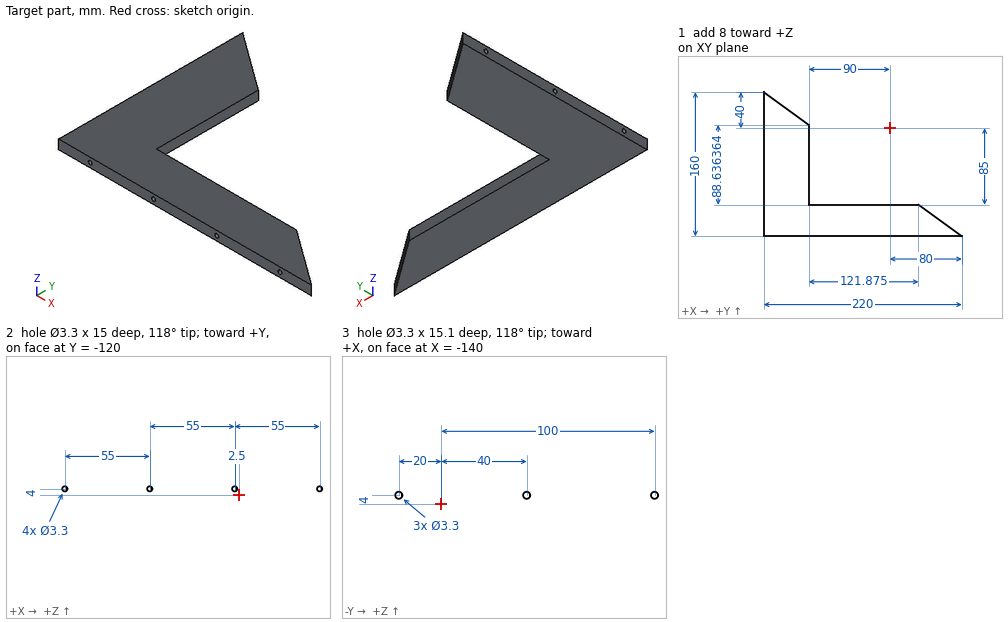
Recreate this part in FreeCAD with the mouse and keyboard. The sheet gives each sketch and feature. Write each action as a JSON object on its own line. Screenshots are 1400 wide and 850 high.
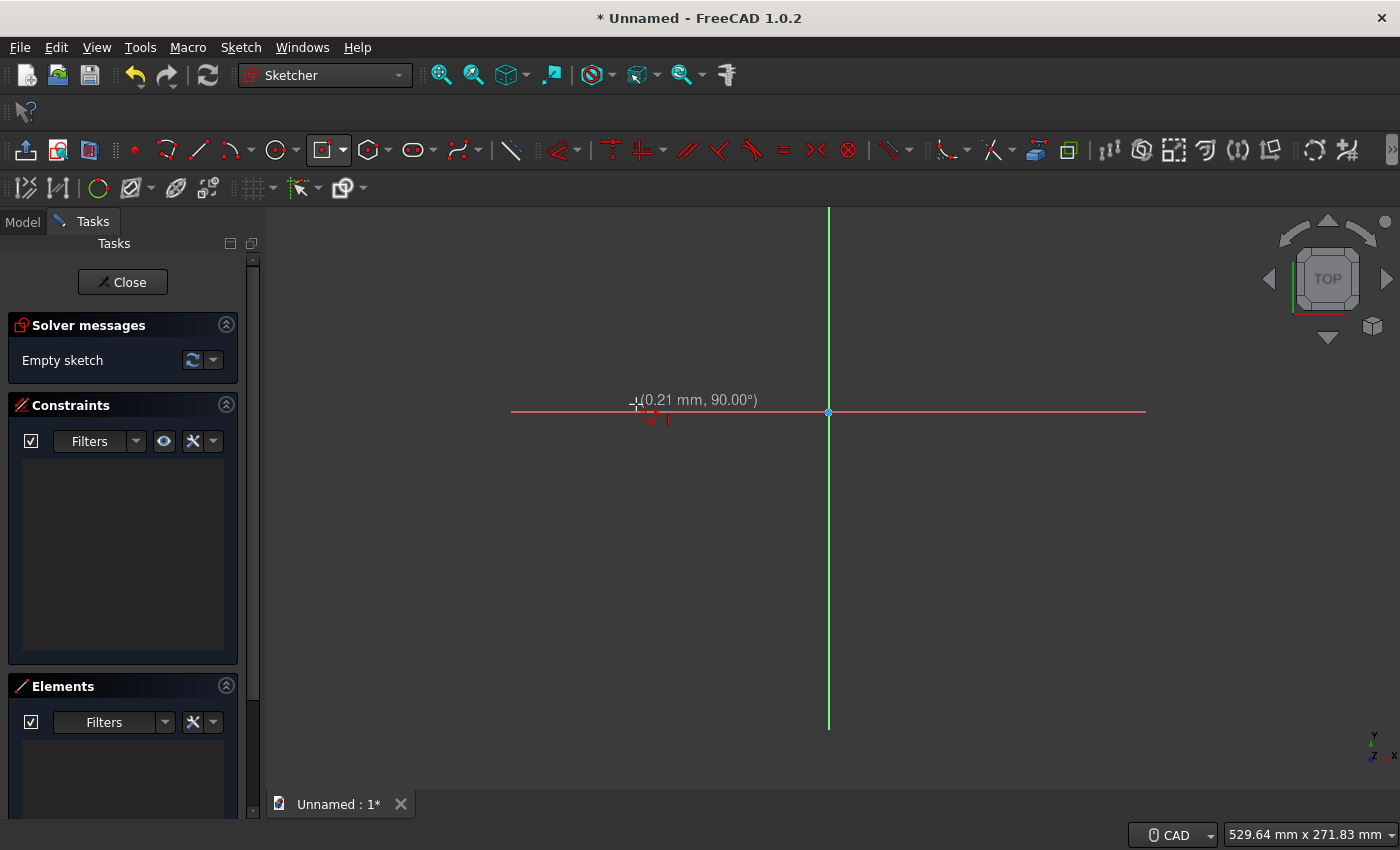
{"action": "left_click", "coordinate": [529, 327]}
{"action": "left_click", "coordinate": [529, 669]}
{"action": "left_click", "coordinate": [1000, 669]}
{"action": "left_click", "coordinate": [897, 594]}
{"action": "left_click", "coordinate": [636, 594]}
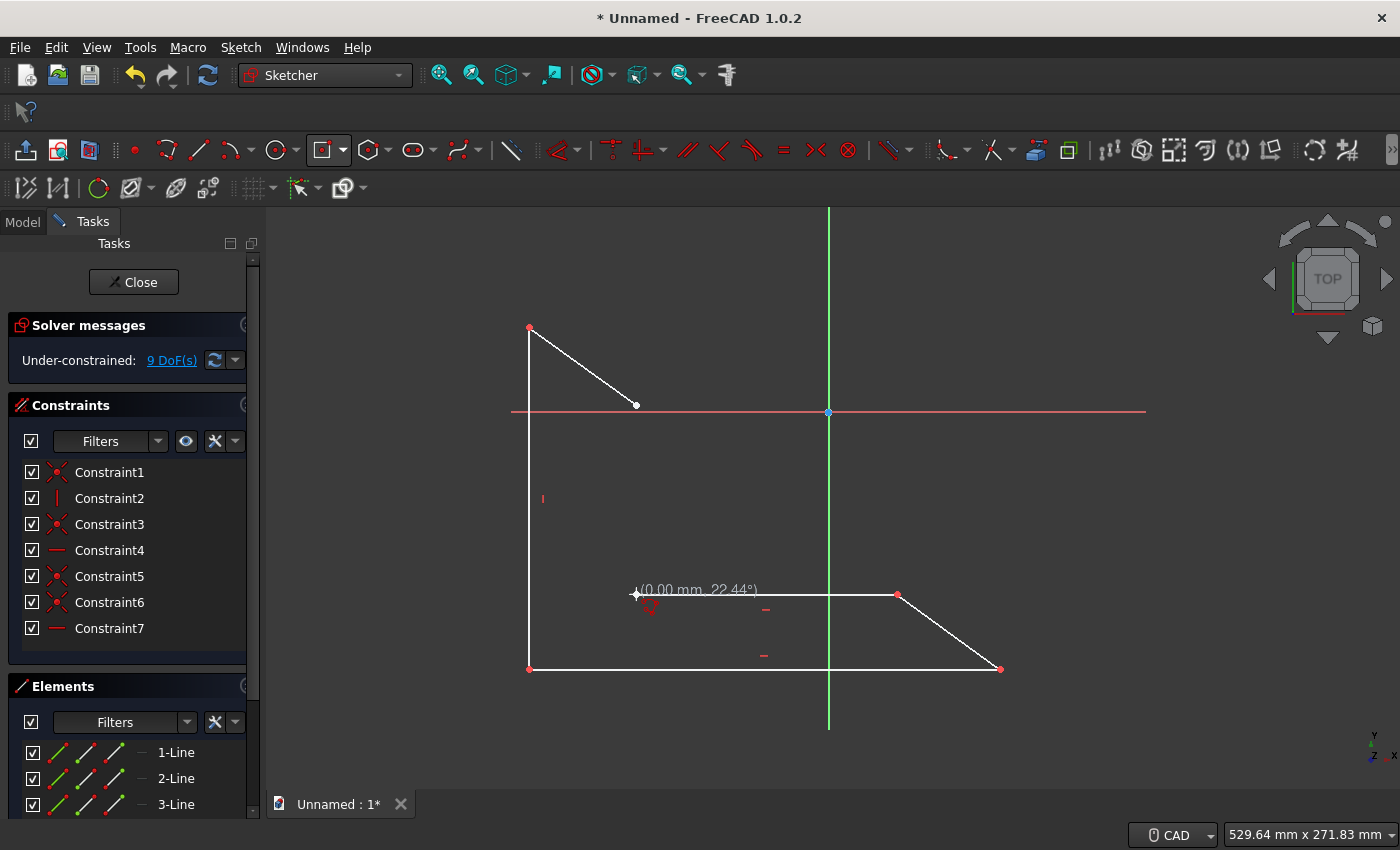
{"action": "scroll", "coordinate": [636, 404], "scroll_direction": "up", "scroll_amount": 4}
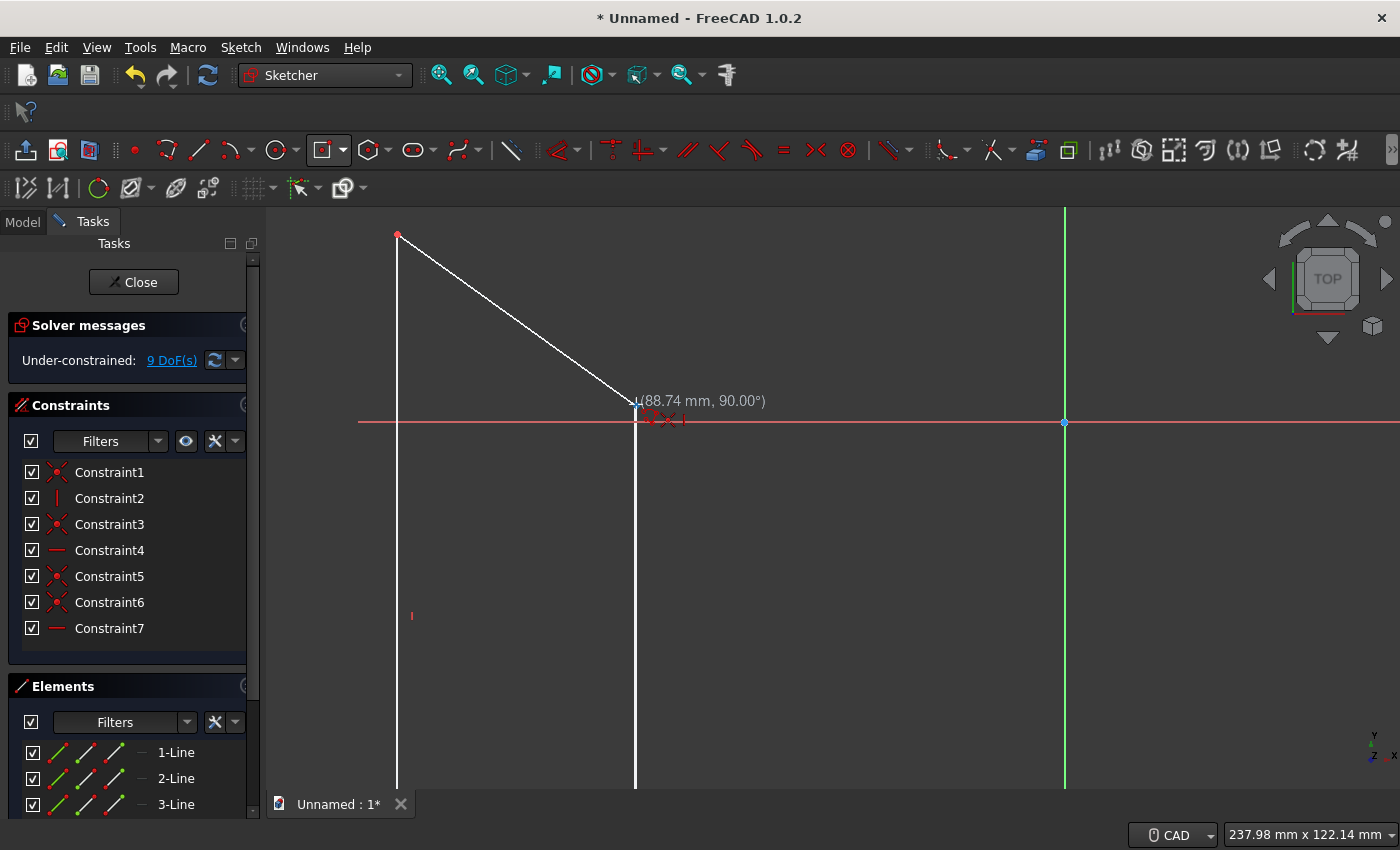
{"action": "left_click", "coordinate": [636, 406]}
{"action": "key", "text": "Escape"}
{"action": "key", "text": "Escape"}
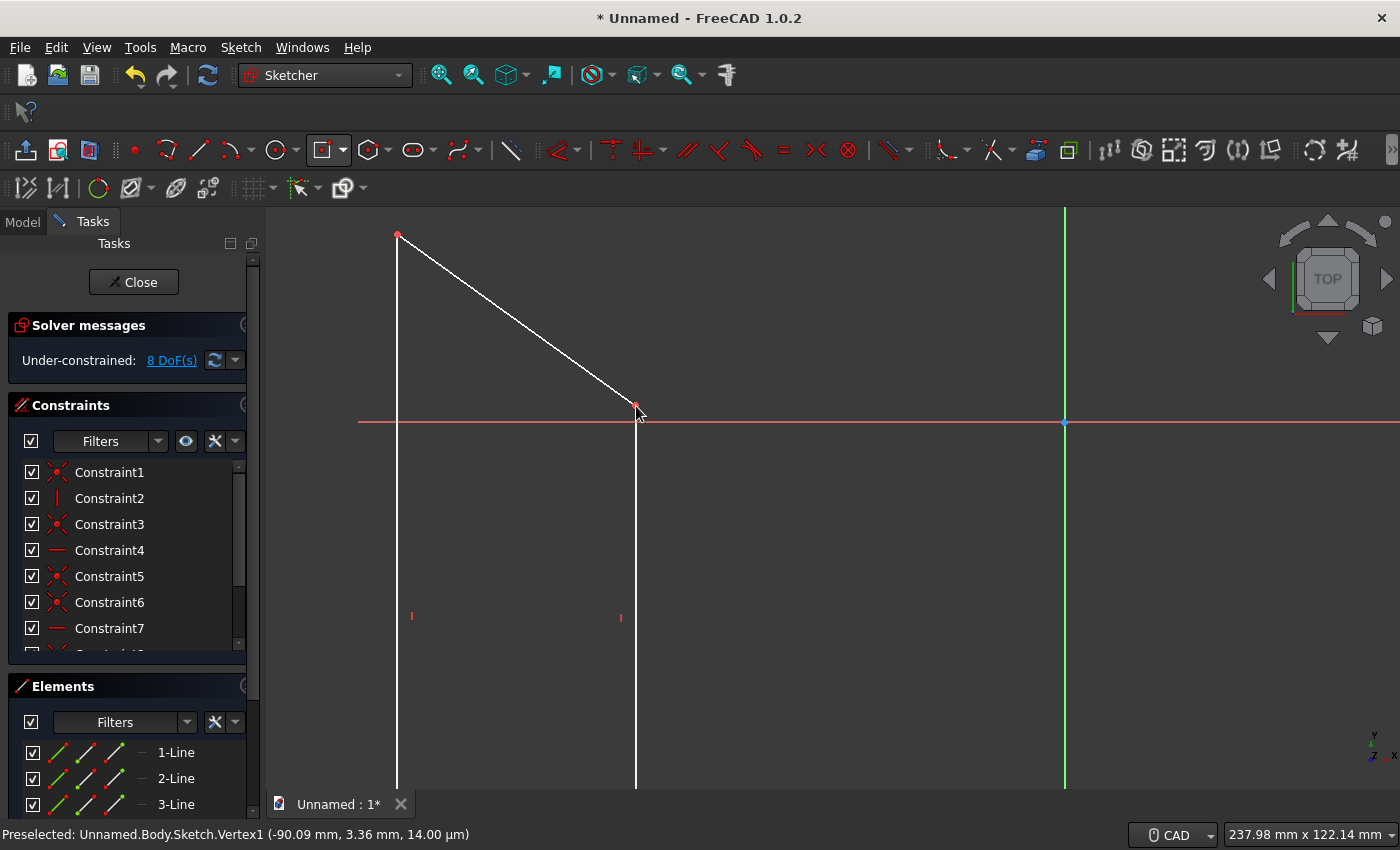
{"action": "key", "text": "d"}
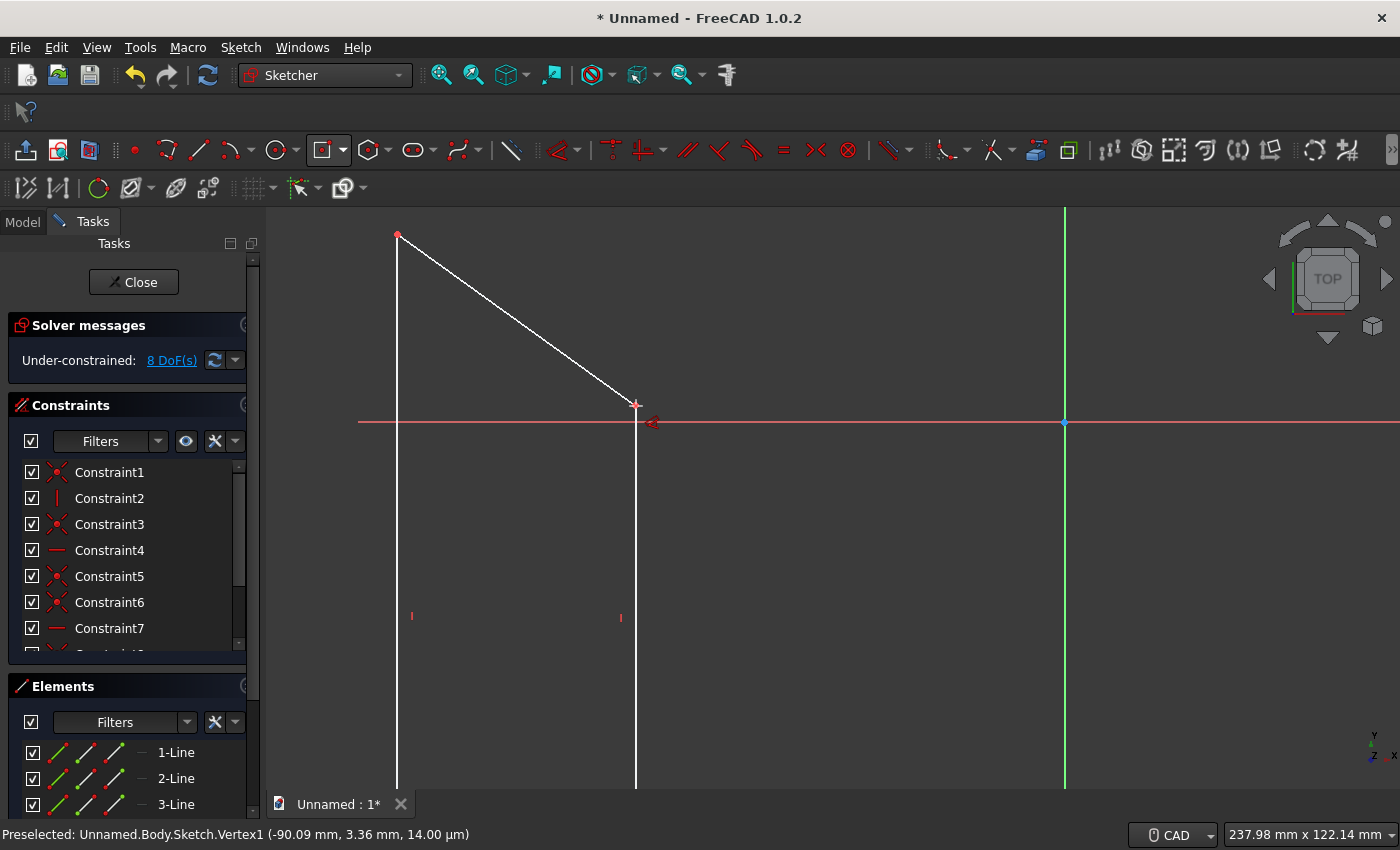
{"action": "left_click", "coordinate": [397, 463]}
{"action": "left_click", "coordinate": [363, 498]}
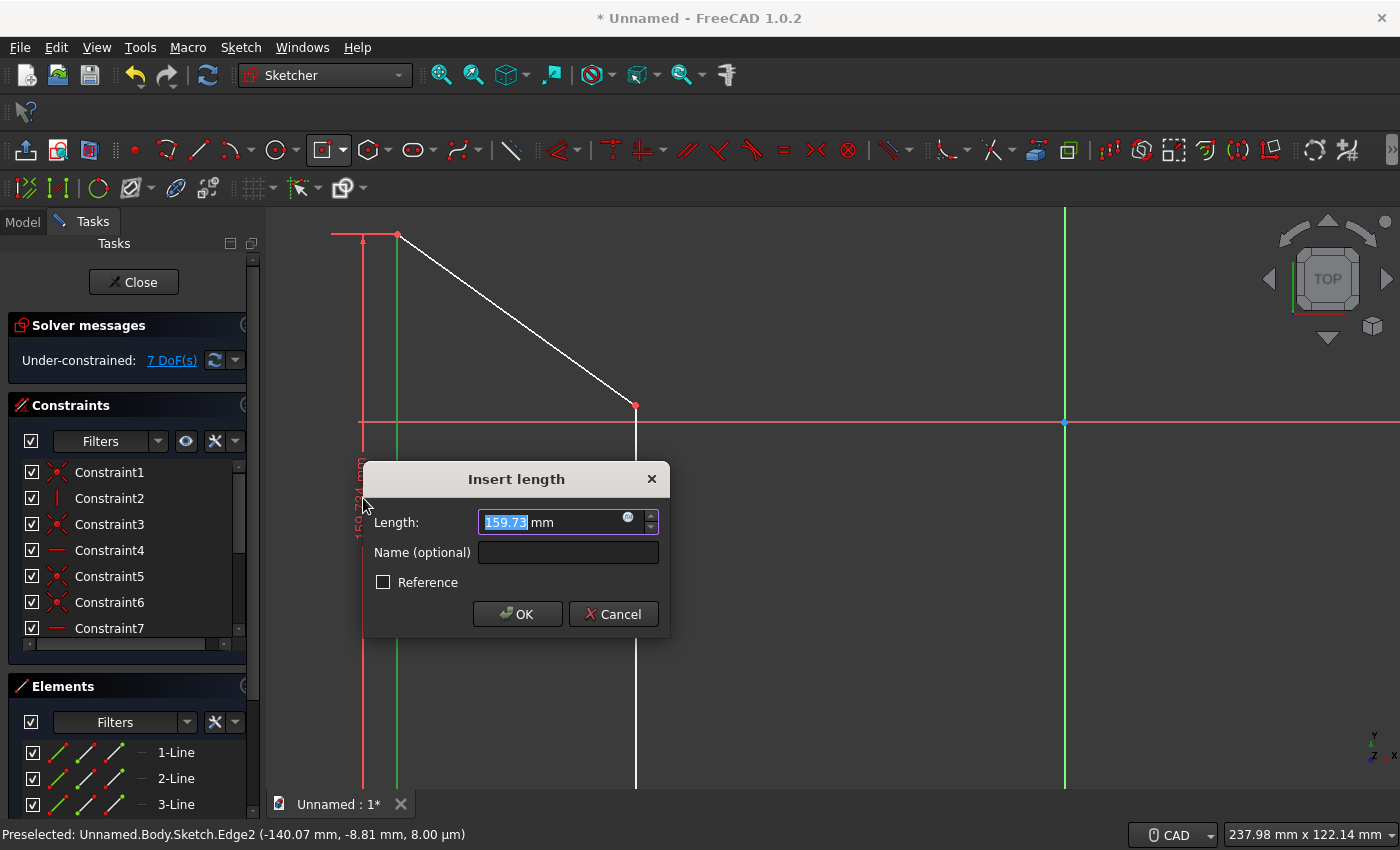
{"action": "type", "text": "160"}
{"action": "key", "text": "Return"}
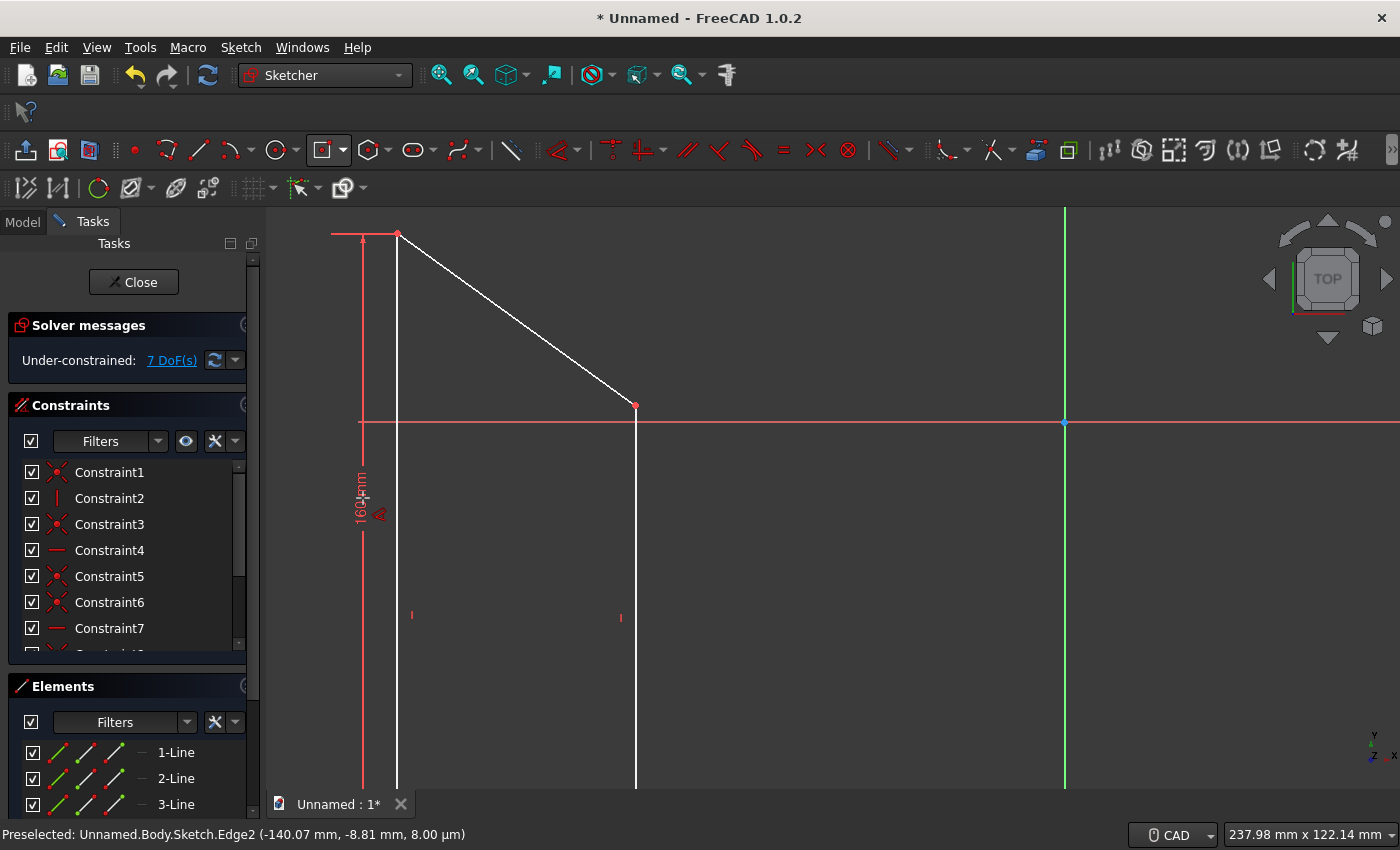
{"action": "scroll", "coordinate": [636, 404], "scroll_direction": "down", "scroll_amount": 4}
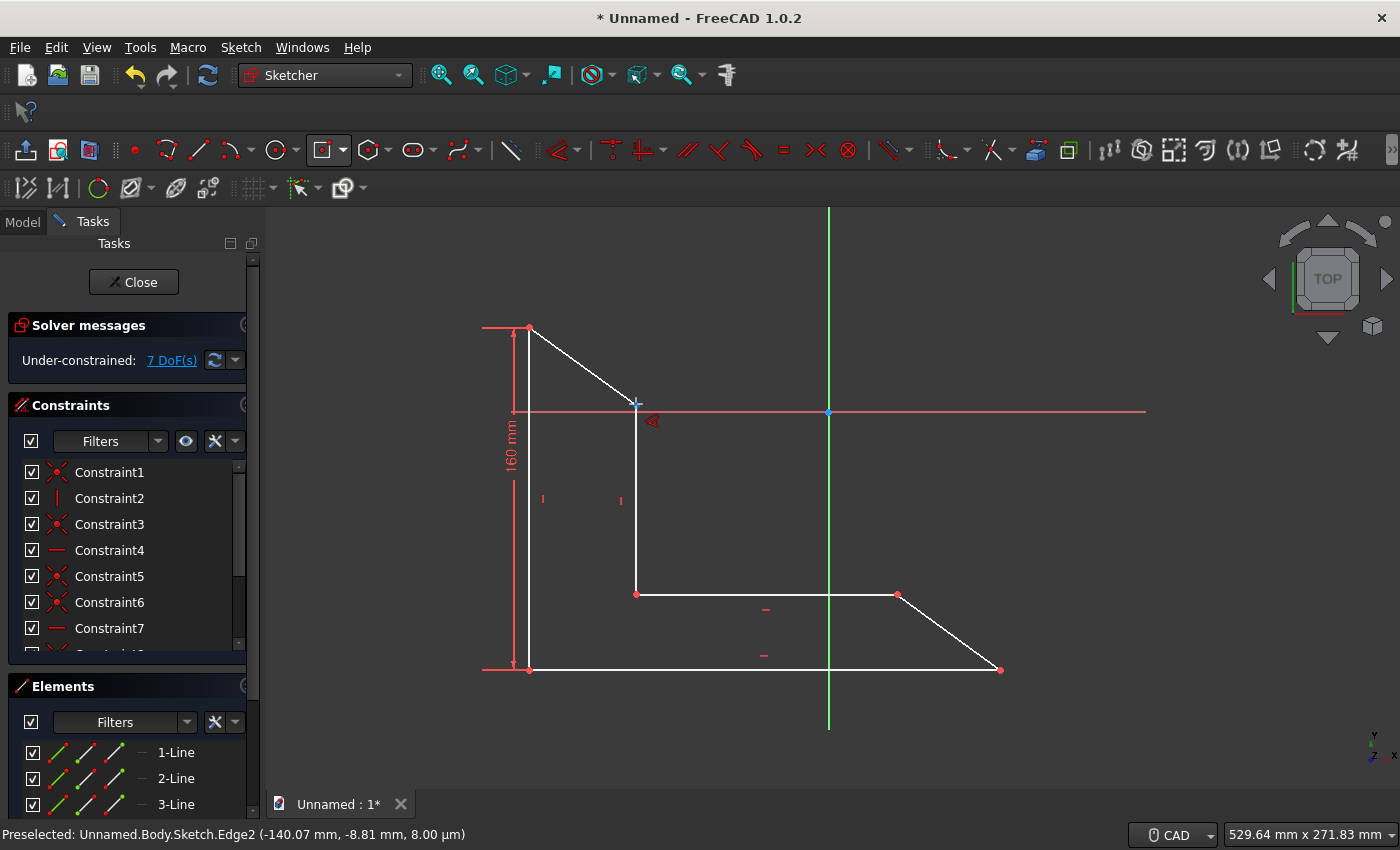
{"action": "left_click", "coordinate": [670, 670]}
{"action": "left_click", "coordinate": [765, 704]}